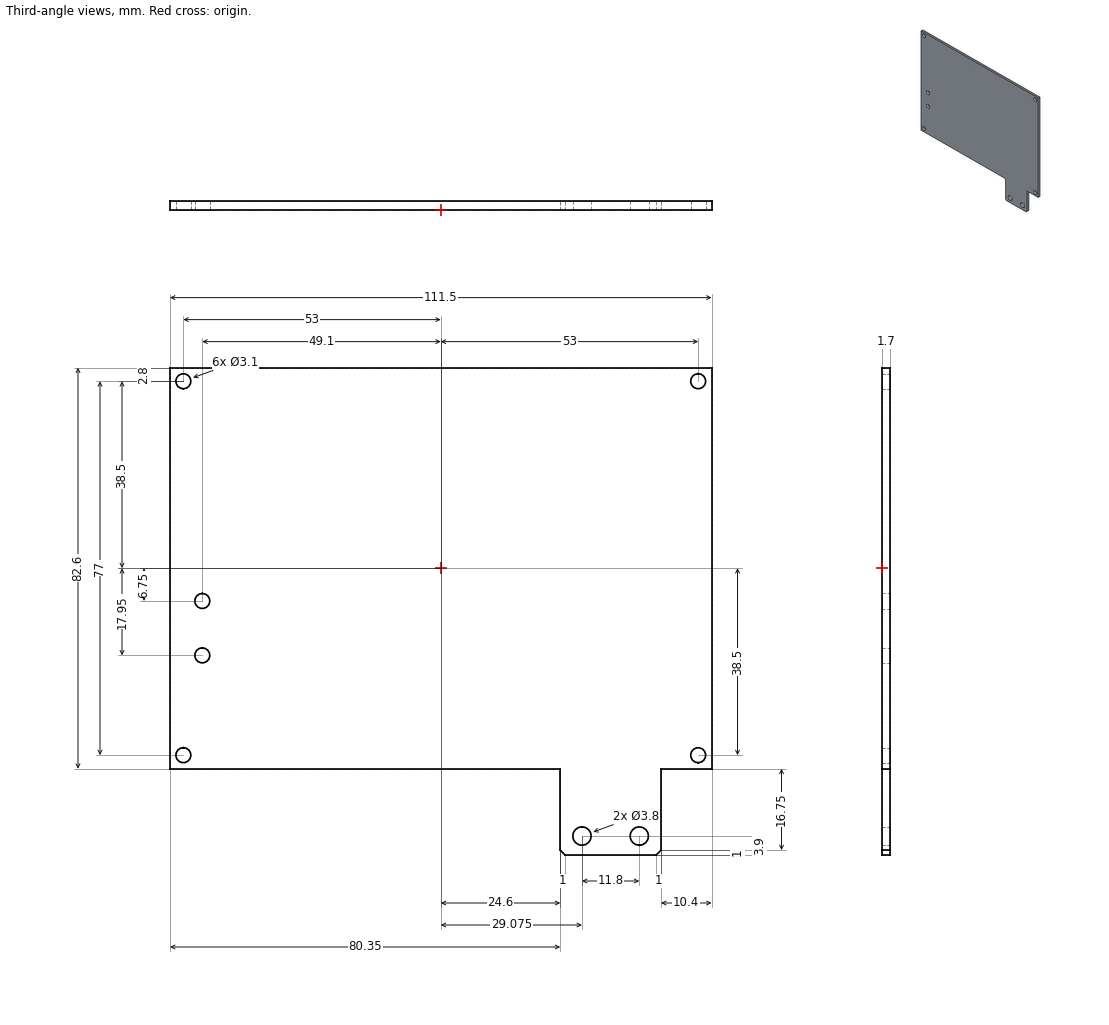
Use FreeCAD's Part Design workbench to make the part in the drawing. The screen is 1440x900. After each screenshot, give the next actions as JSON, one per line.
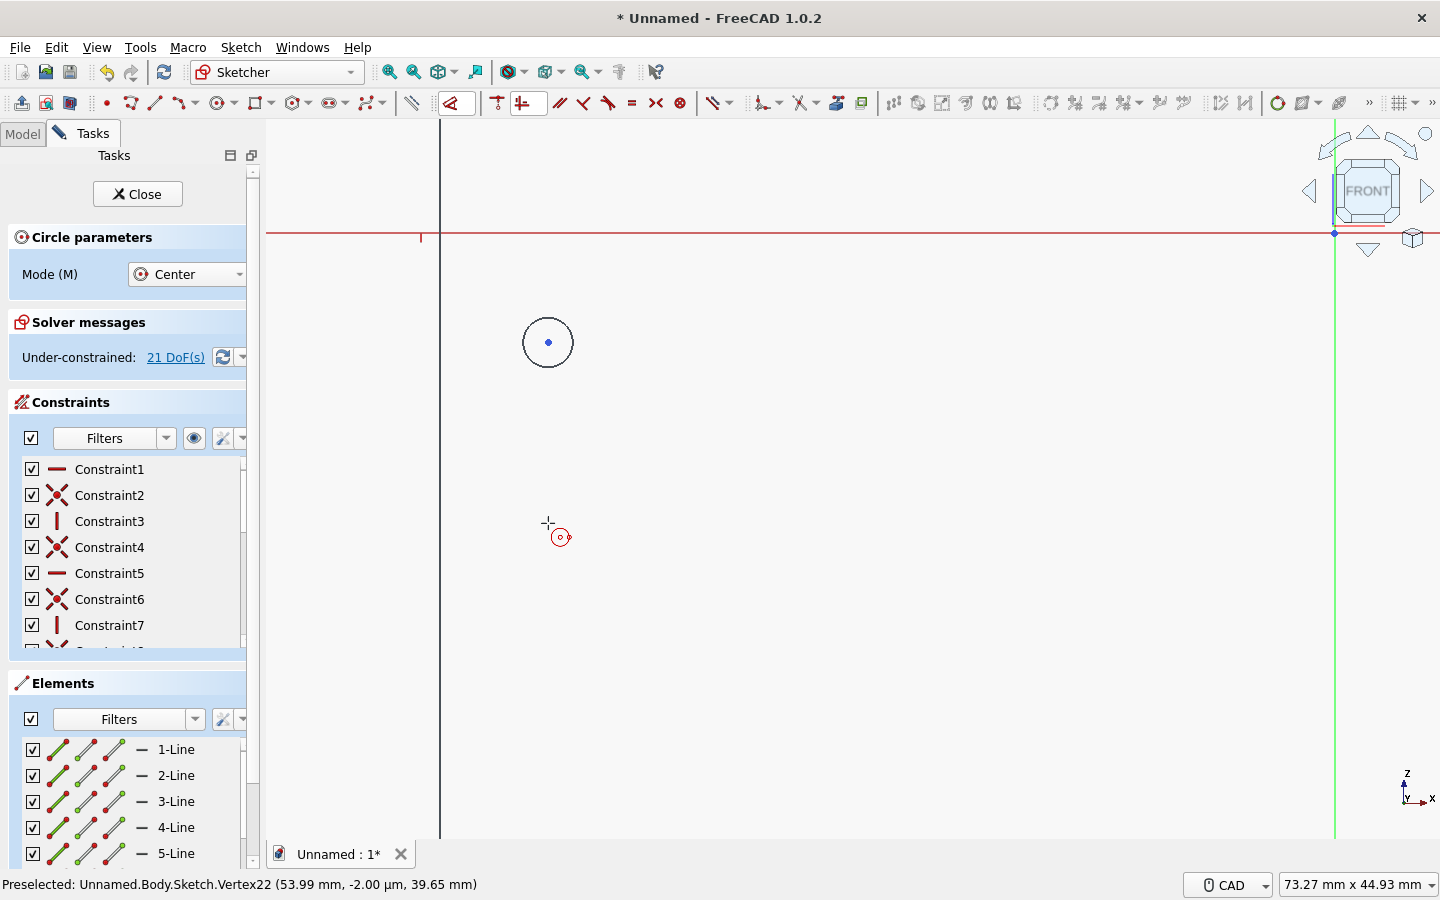
{"action": "left_click", "coordinate": [548, 521]}
{"action": "left_click", "coordinate": [566, 504]}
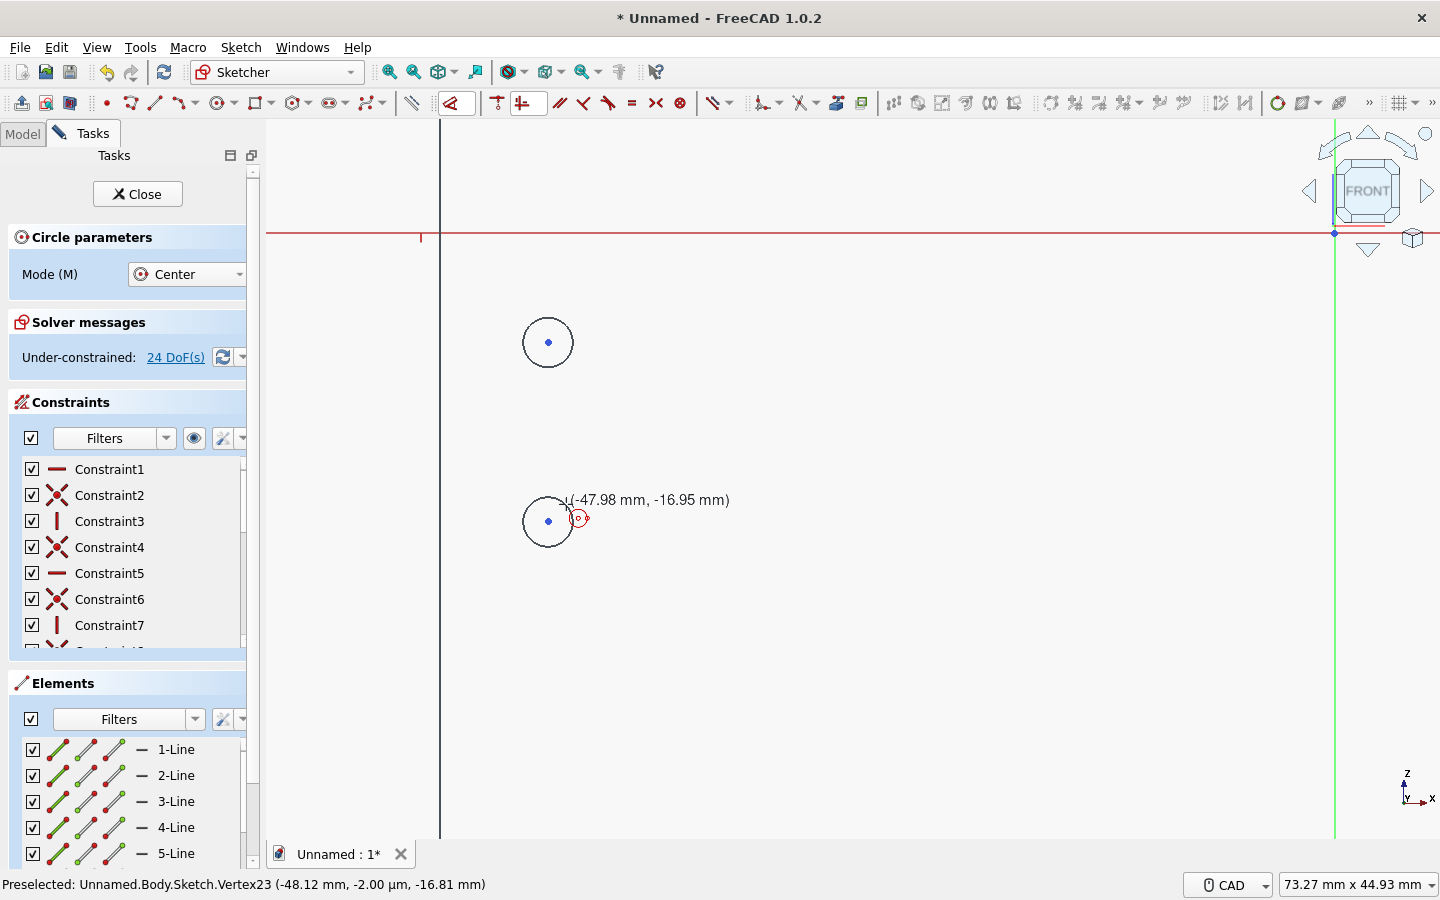
{"action": "scroll", "coordinate": [547, 524], "scroll_direction": "down", "scroll_amount": 6}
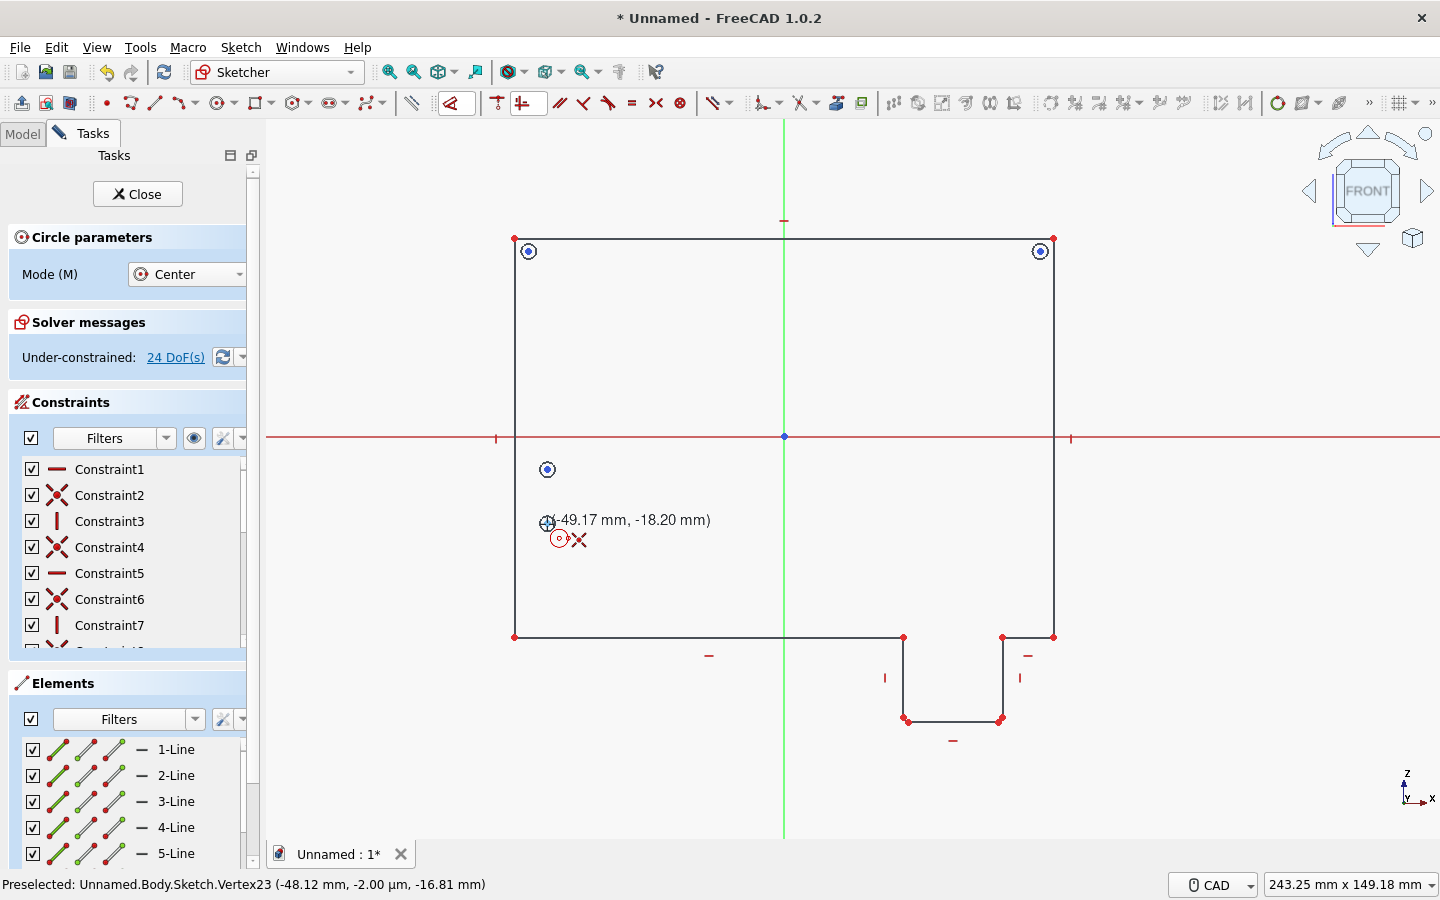
{"action": "scroll", "coordinate": [529, 623], "scroll_direction": "up", "scroll_amount": 6}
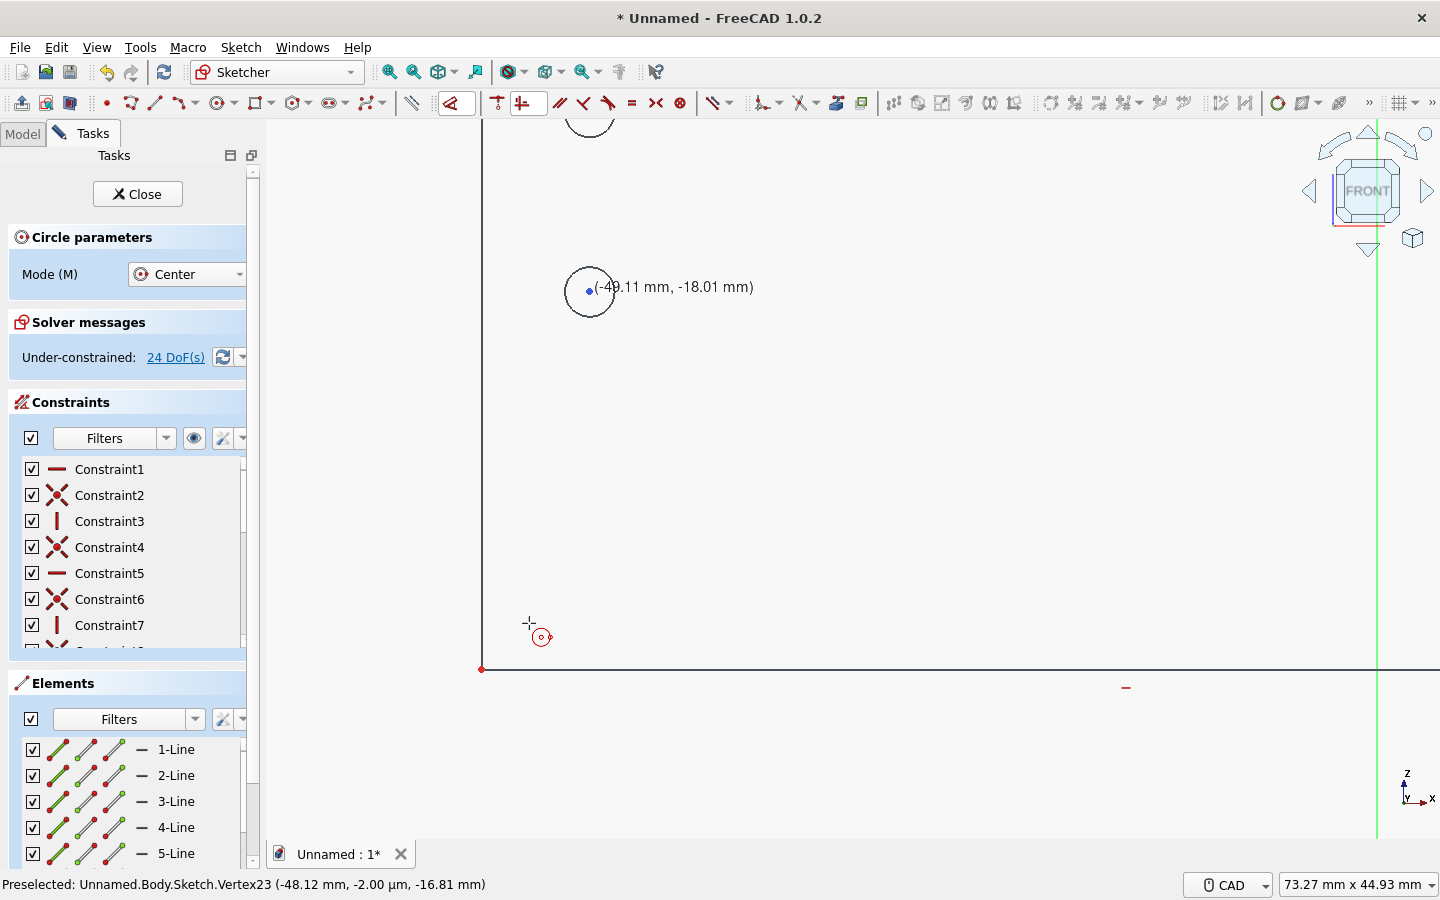
{"action": "left_click", "coordinate": [527, 620]}
{"action": "left_click", "coordinate": [545, 603]}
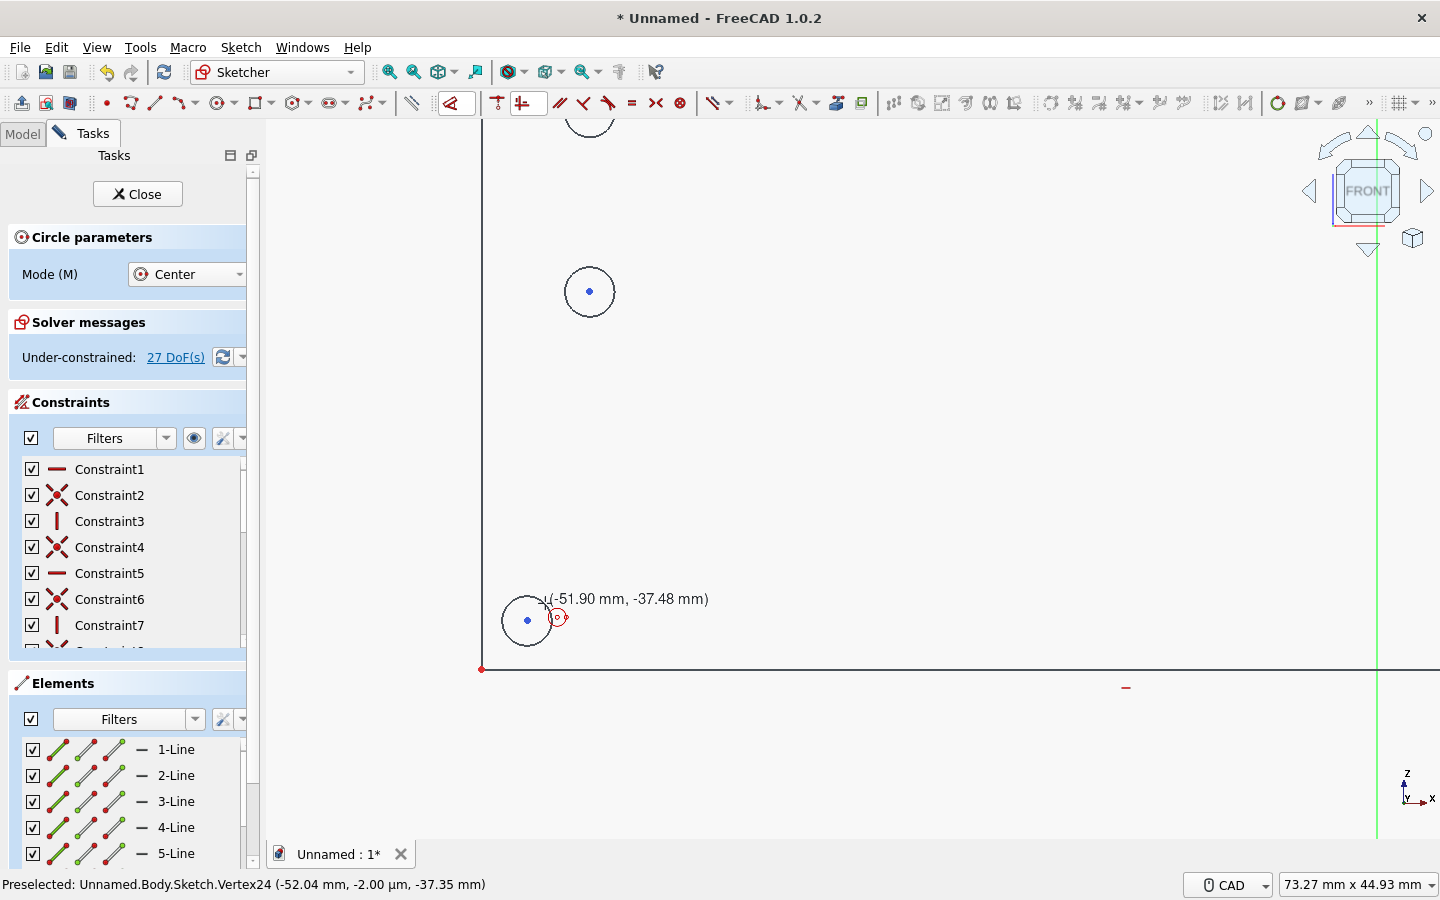
{"action": "scroll", "coordinate": [529, 623], "scroll_direction": "down", "scroll_amount": 6}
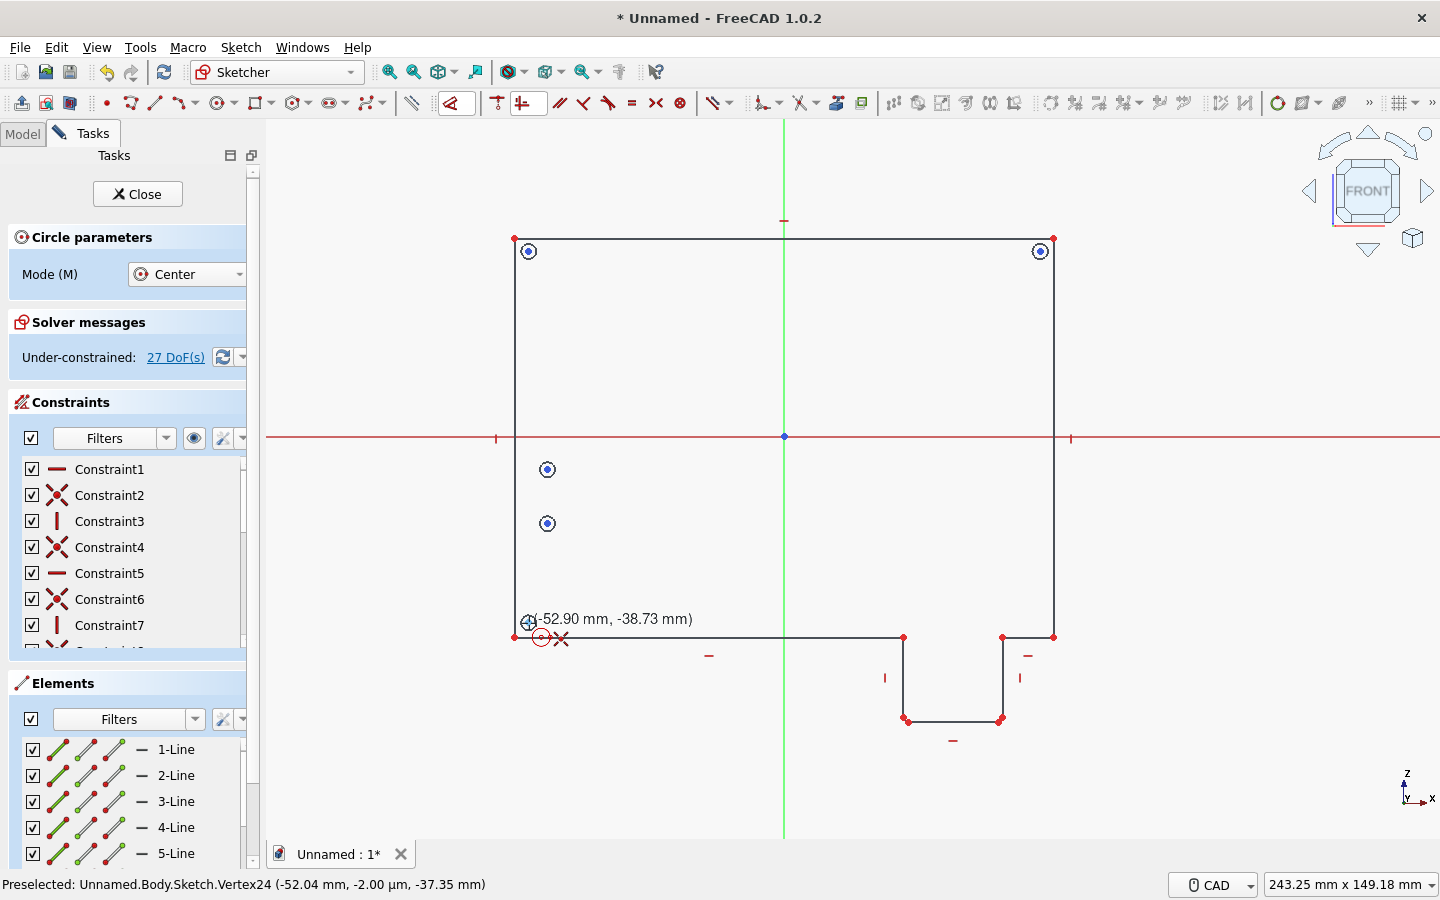
{"action": "scroll", "coordinate": [1040, 623], "scroll_direction": "up", "scroll_amount": 6}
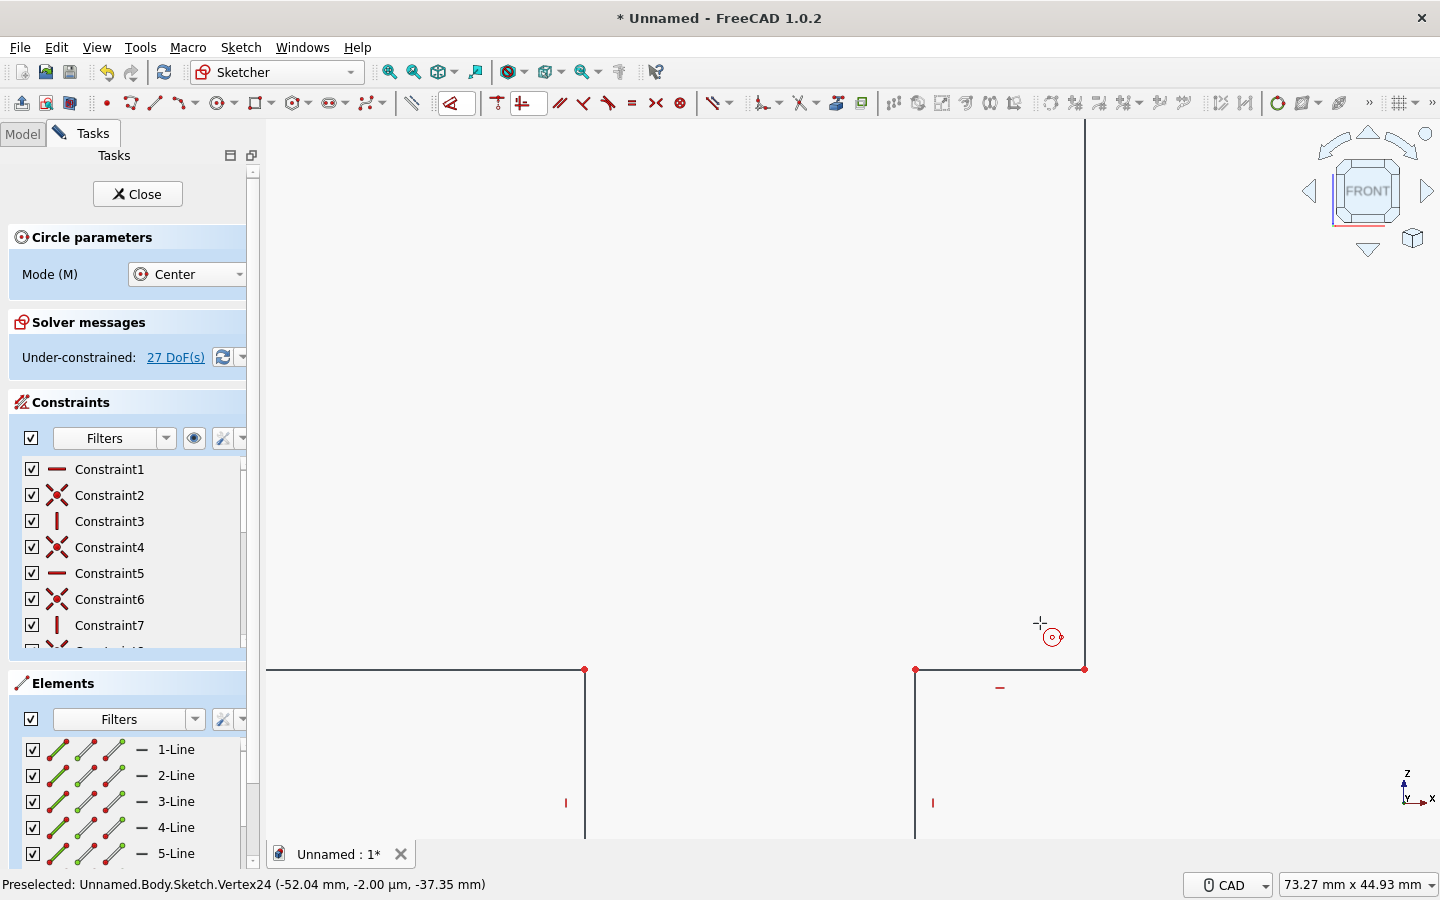
{"action": "left_click", "coordinate": [1039, 620]}
{"action": "left_click", "coordinate": [1057, 603]}